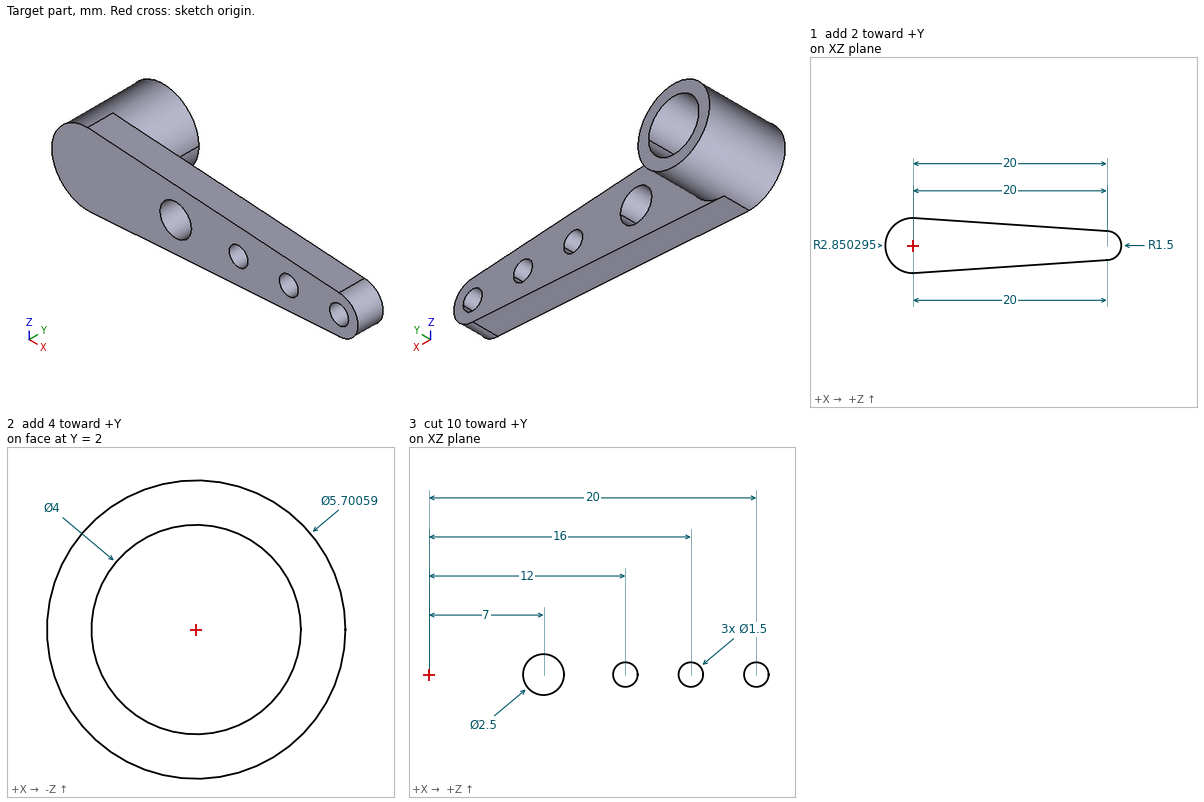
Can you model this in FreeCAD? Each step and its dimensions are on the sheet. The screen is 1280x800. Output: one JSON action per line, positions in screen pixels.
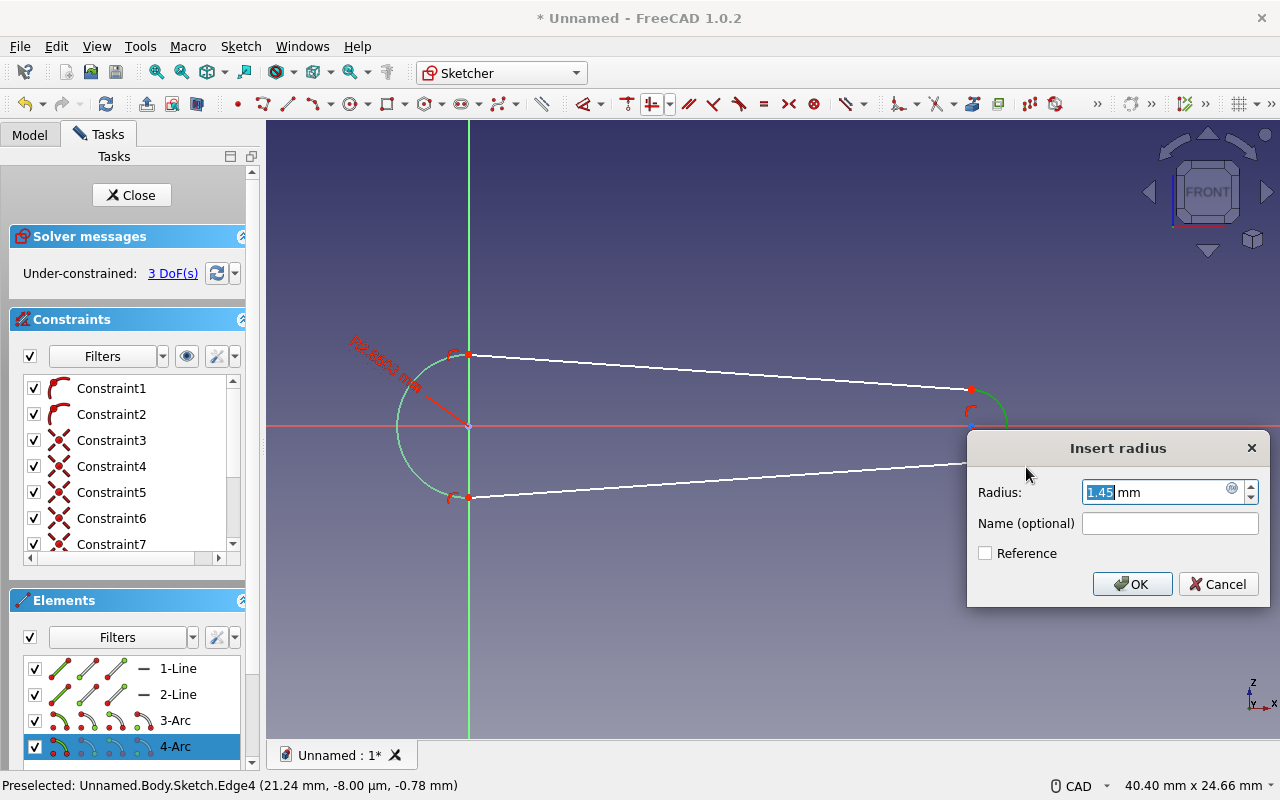
{"action": "type", "text": "1.5"}
{"action": "key", "text": "Return"}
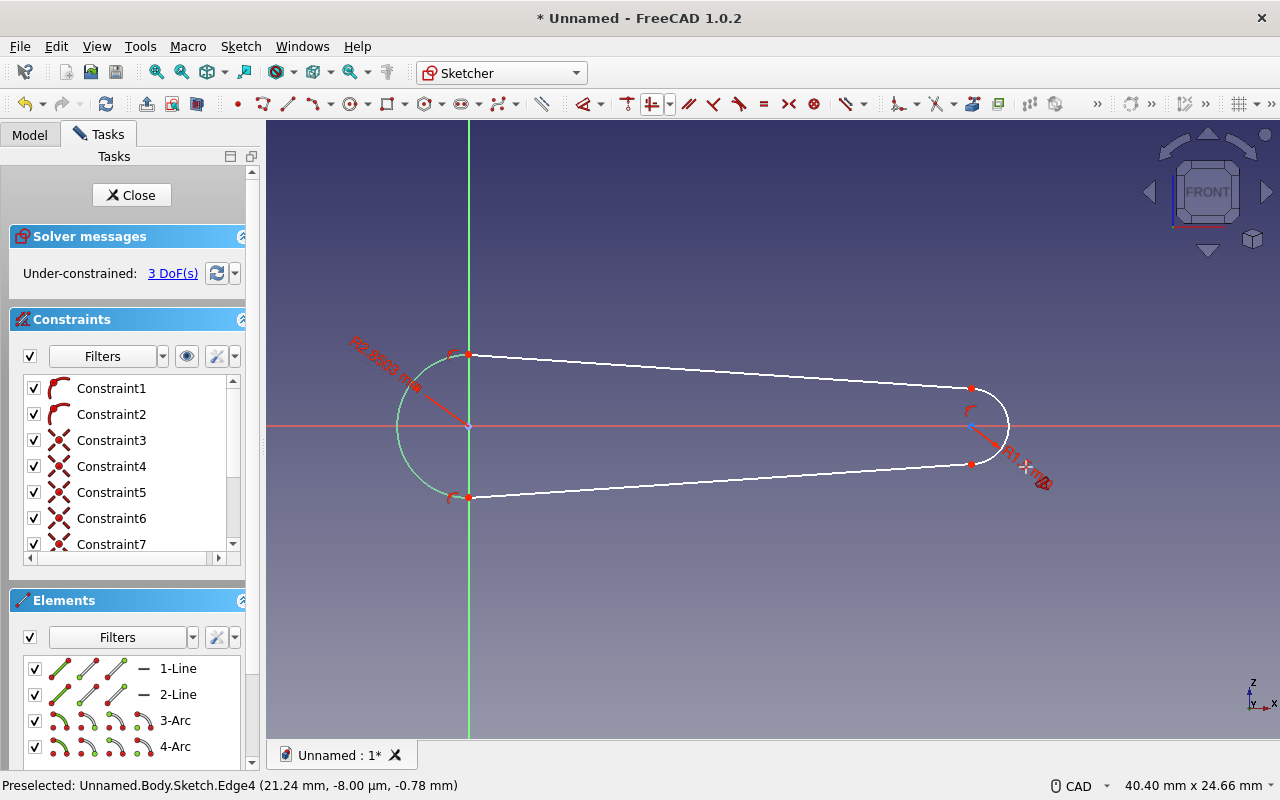
{"action": "left_click", "coordinate": [971, 464]}
{"action": "left_click", "coordinate": [720, 498]}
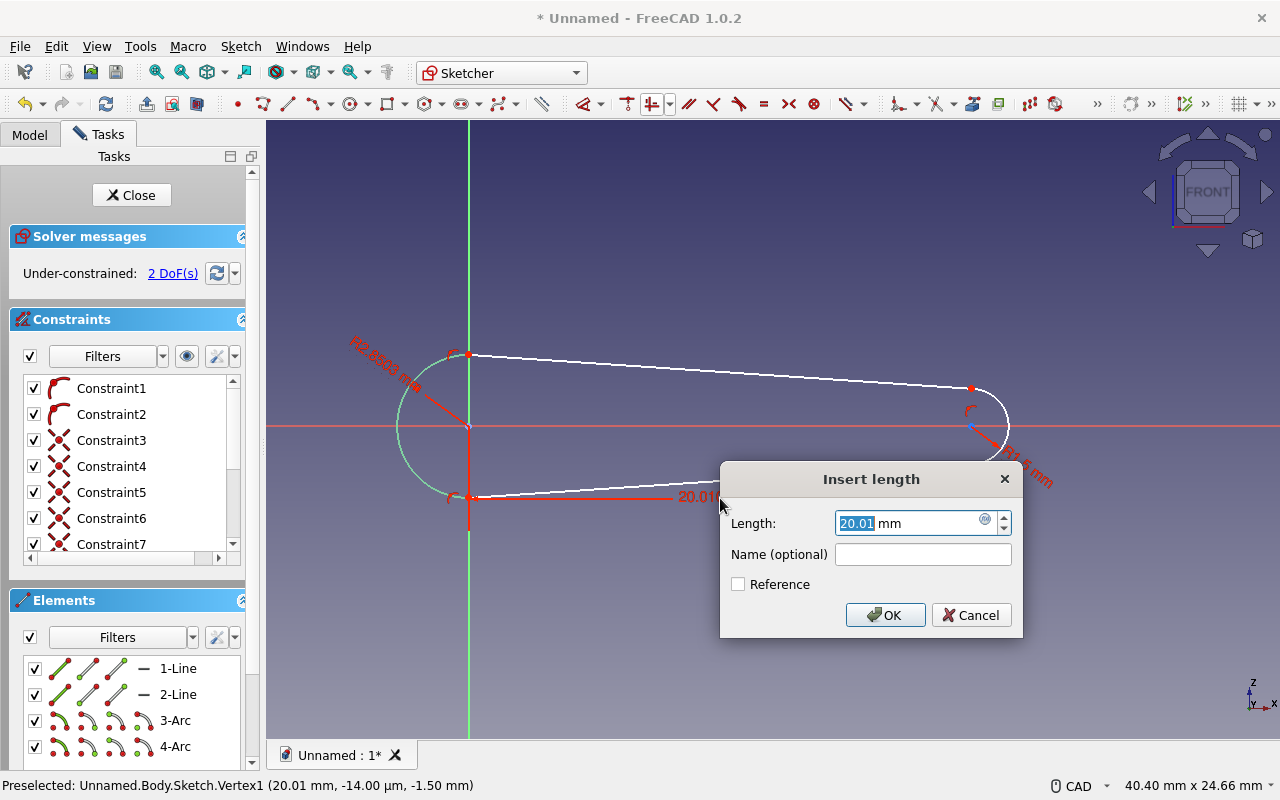
{"action": "type", "text": "20"}
{"action": "key", "text": "Return"}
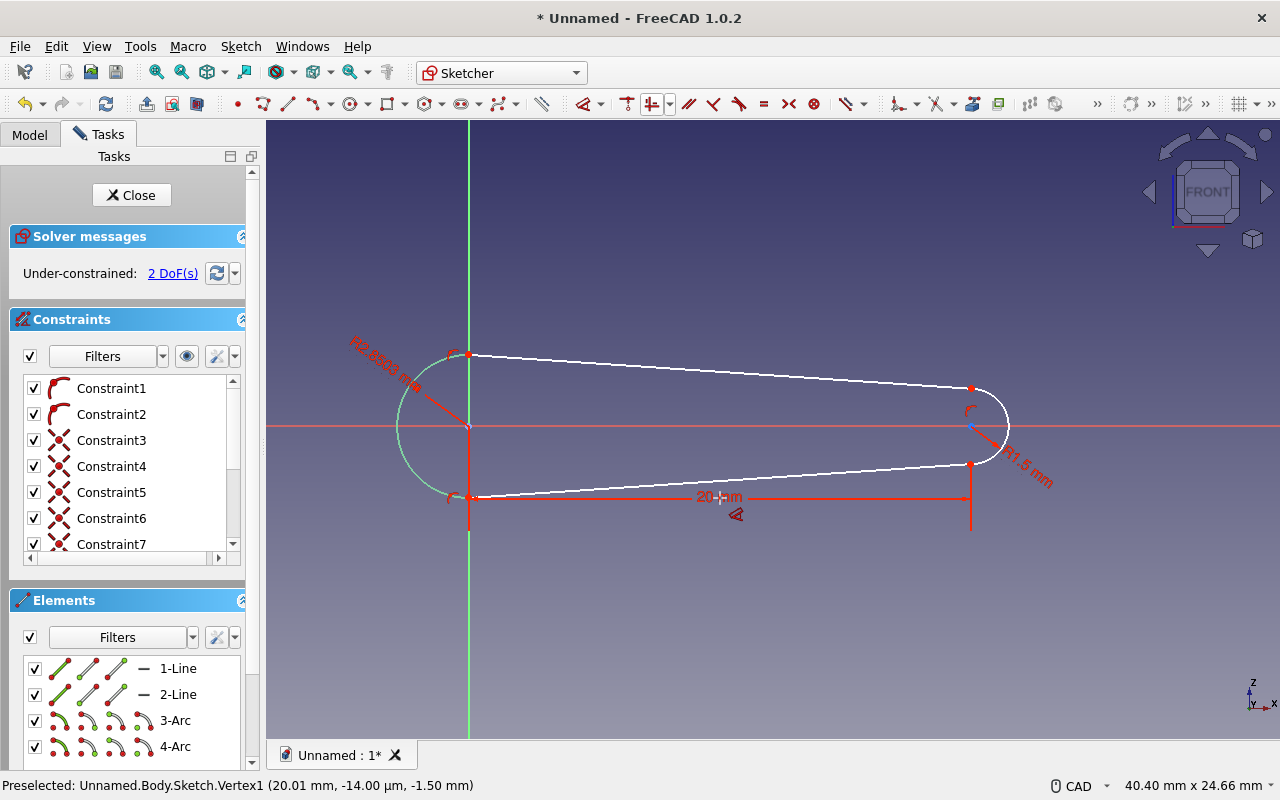
{"action": "left_click", "coordinate": [971, 389]}
{"action": "left_click", "coordinate": [720, 355]}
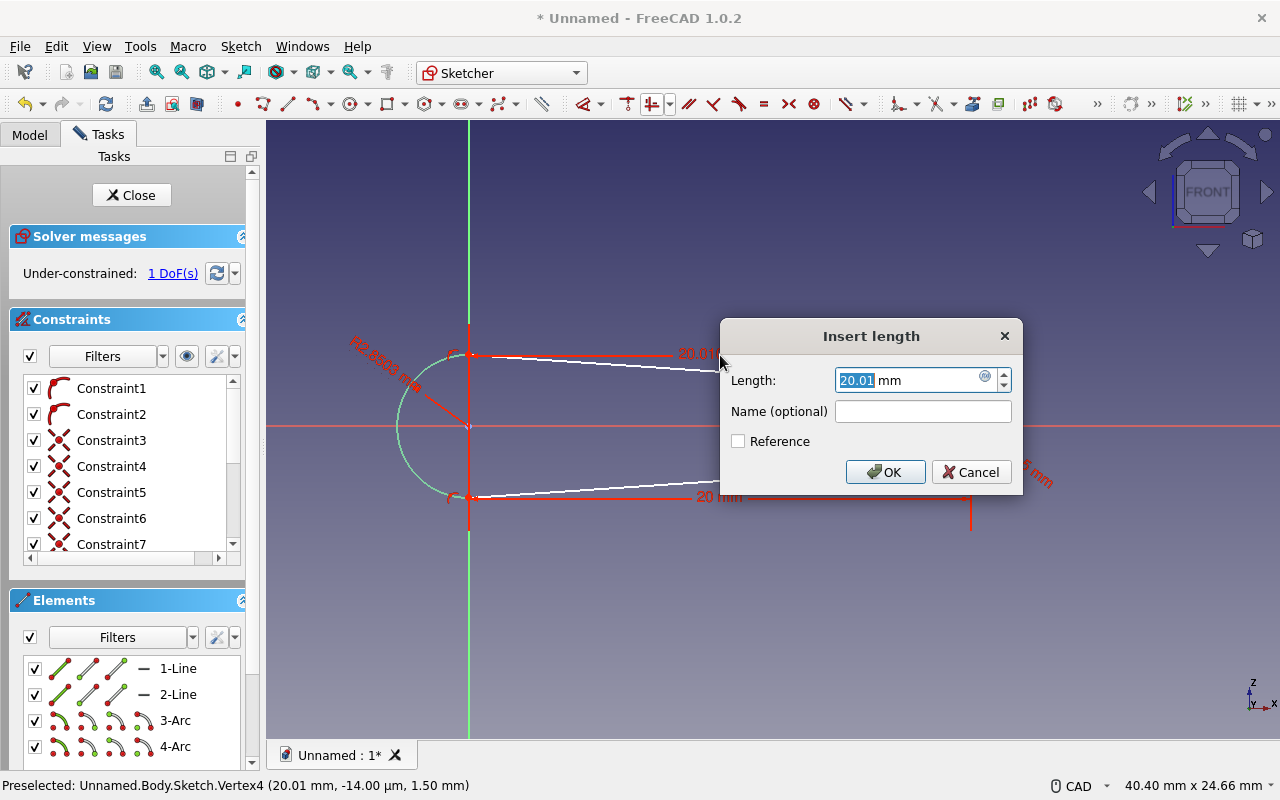
{"action": "type", "text": "20"}
{"action": "key", "text": "Return"}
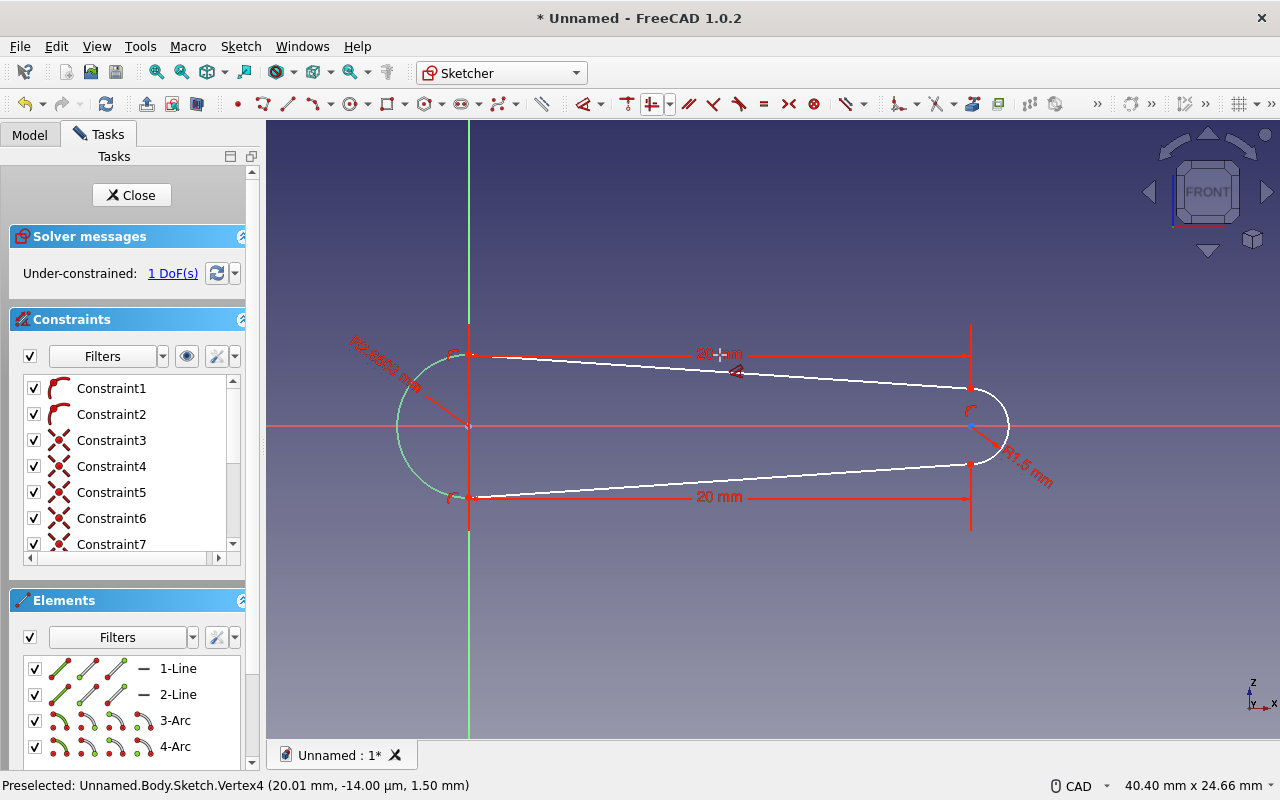
{"action": "left_click", "coordinate": [971, 426]}
{"action": "left_click", "coordinate": [720, 460]}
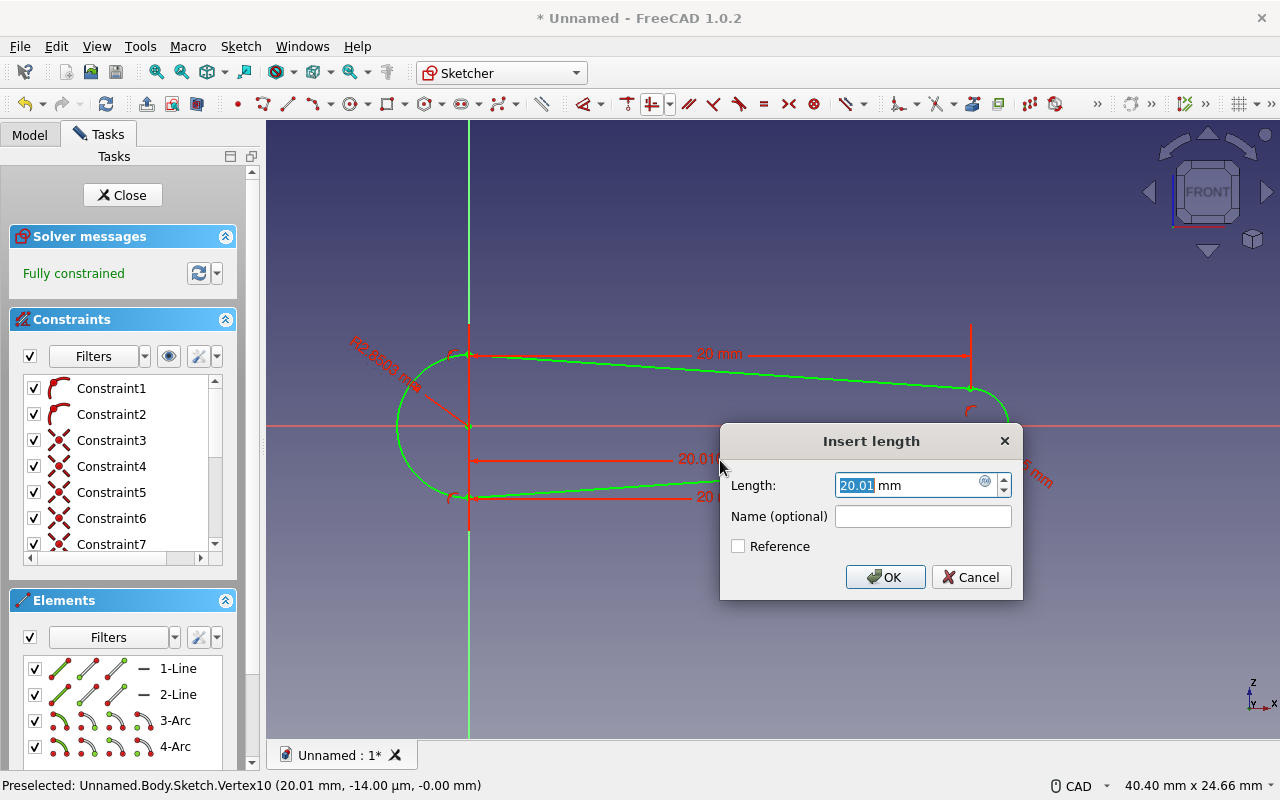
{"action": "type", "text": "20"}
{"action": "key", "text": "Return"}
{"action": "key", "text": "Escape"}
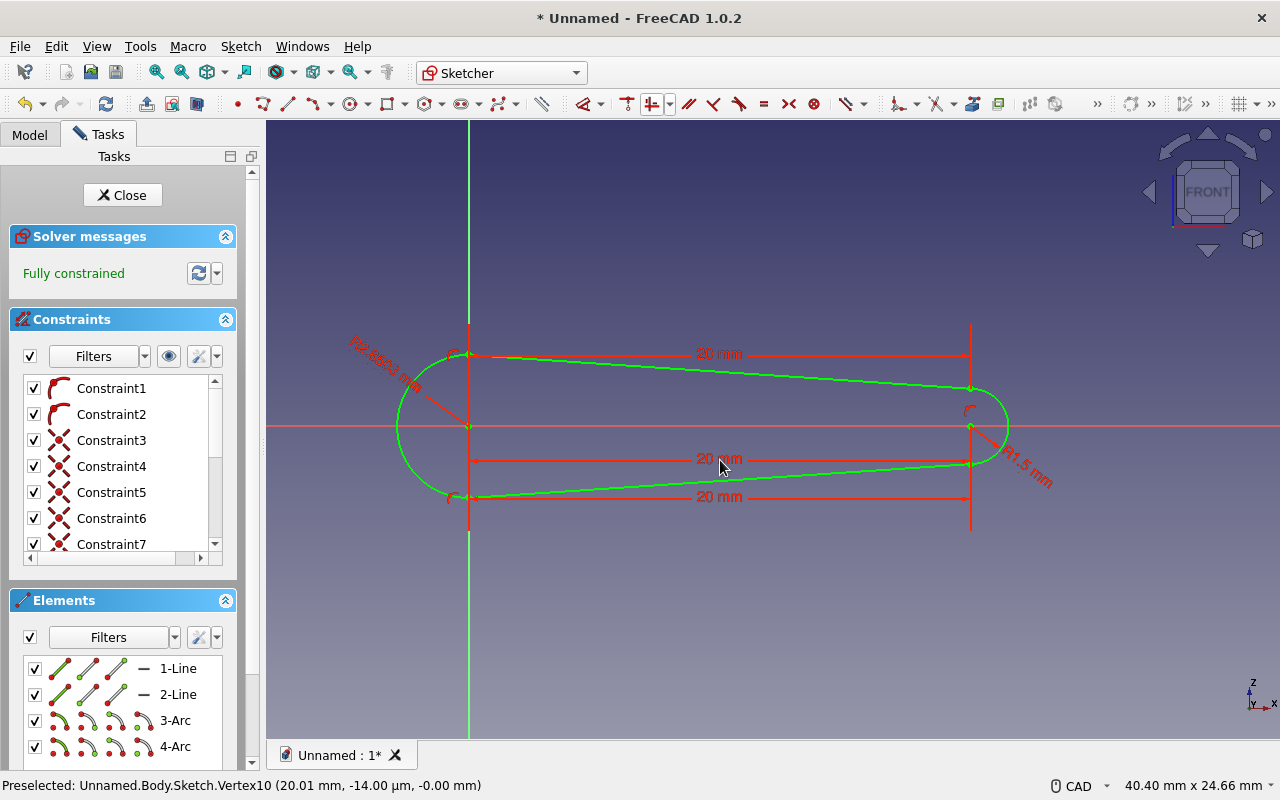
{"action": "left_click", "coordinate": [123, 195]}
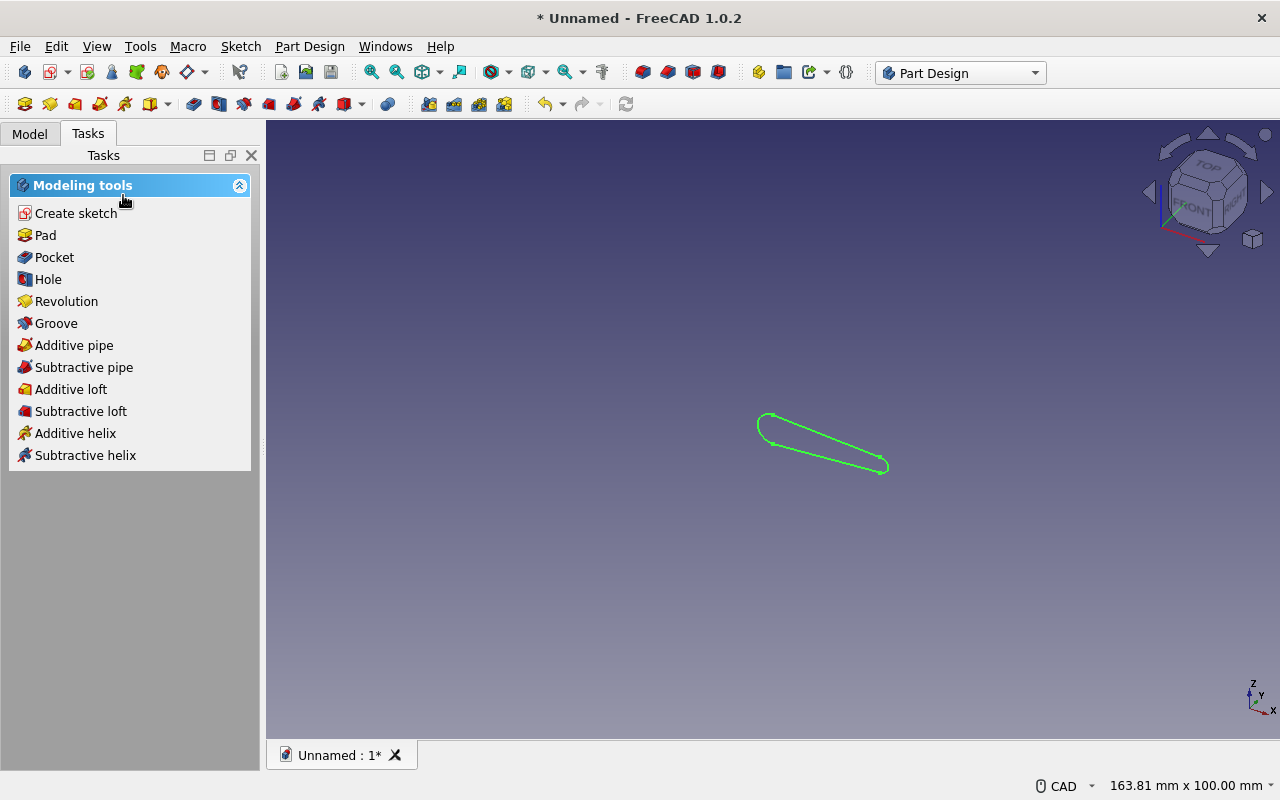
{"action": "left_click", "coordinate": [25, 104]}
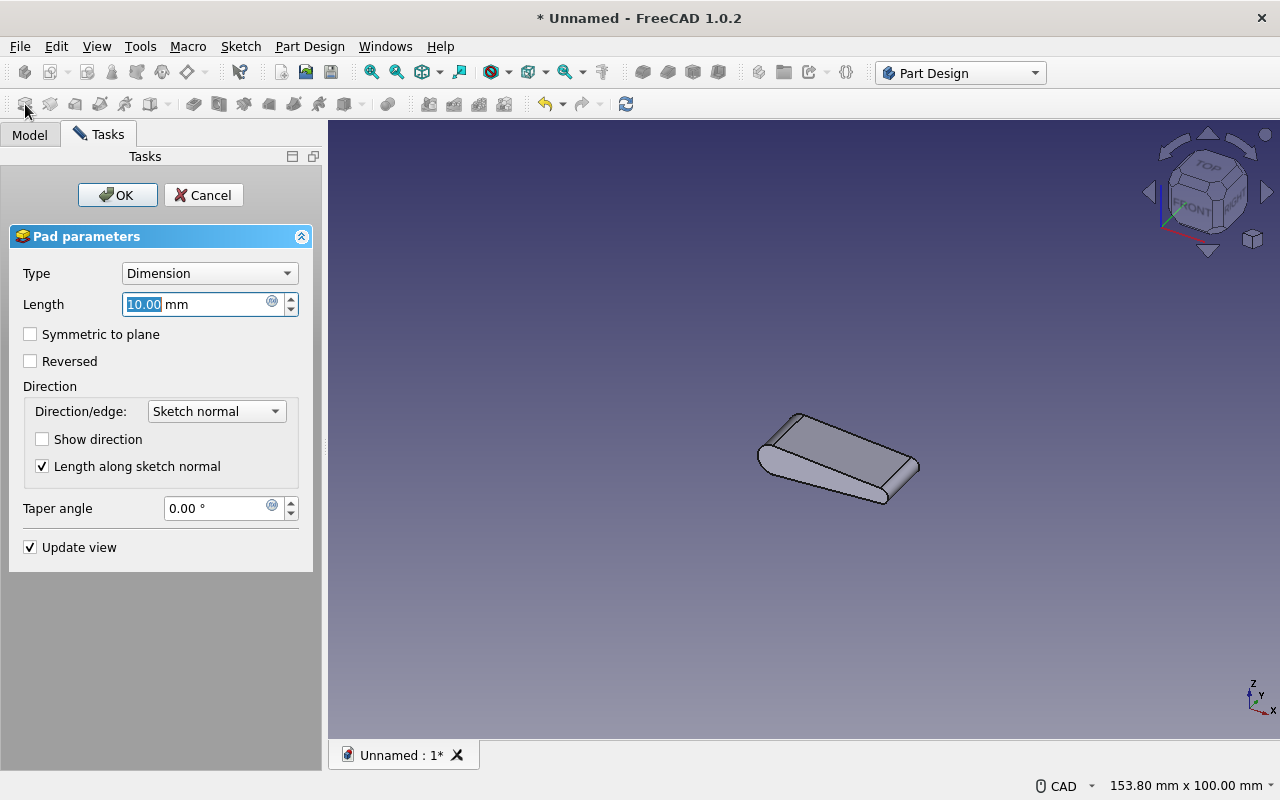
{"action": "type", "text": "2"}
{"action": "key", "text": "Tab"}